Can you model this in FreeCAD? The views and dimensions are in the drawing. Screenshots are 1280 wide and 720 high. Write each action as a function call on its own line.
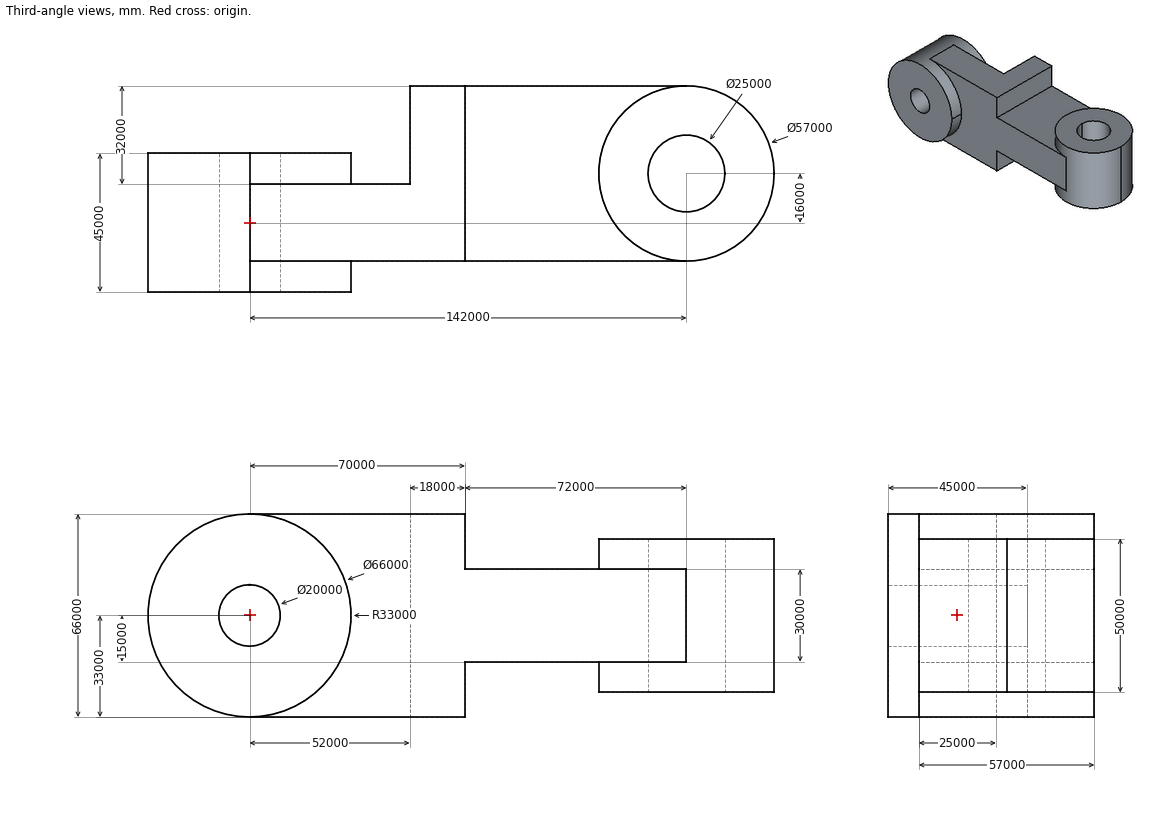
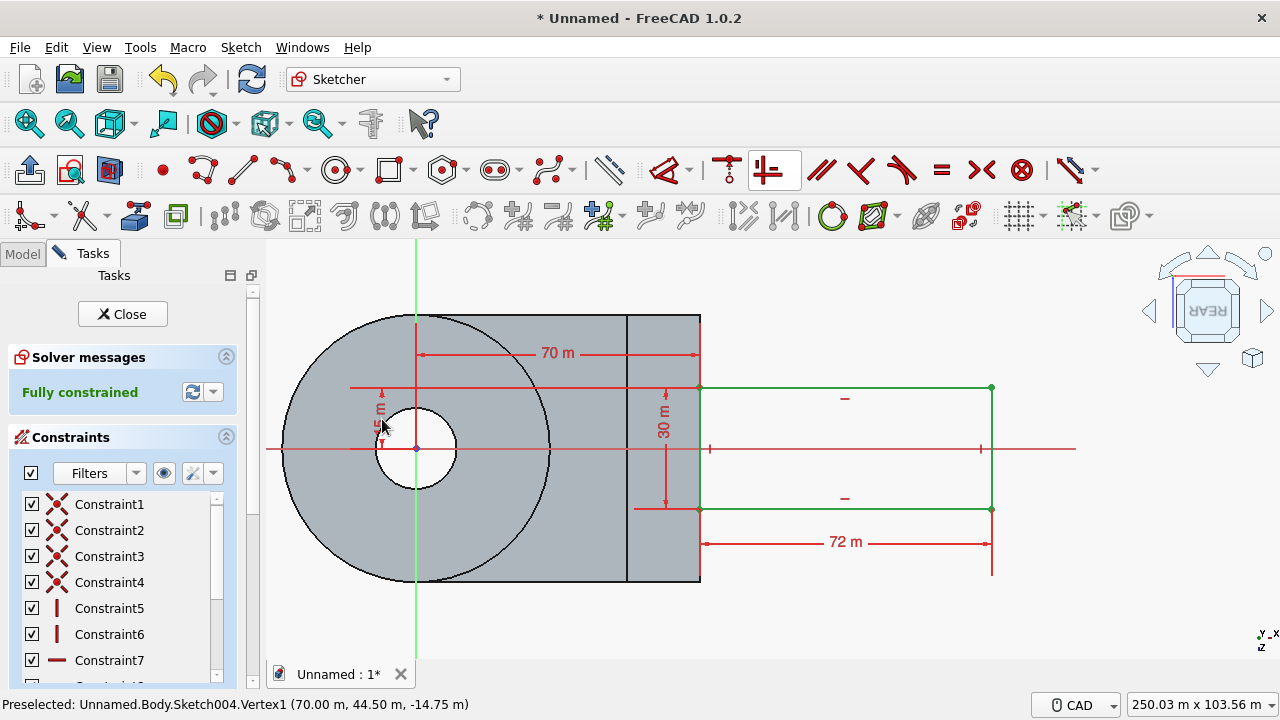
click(123, 314)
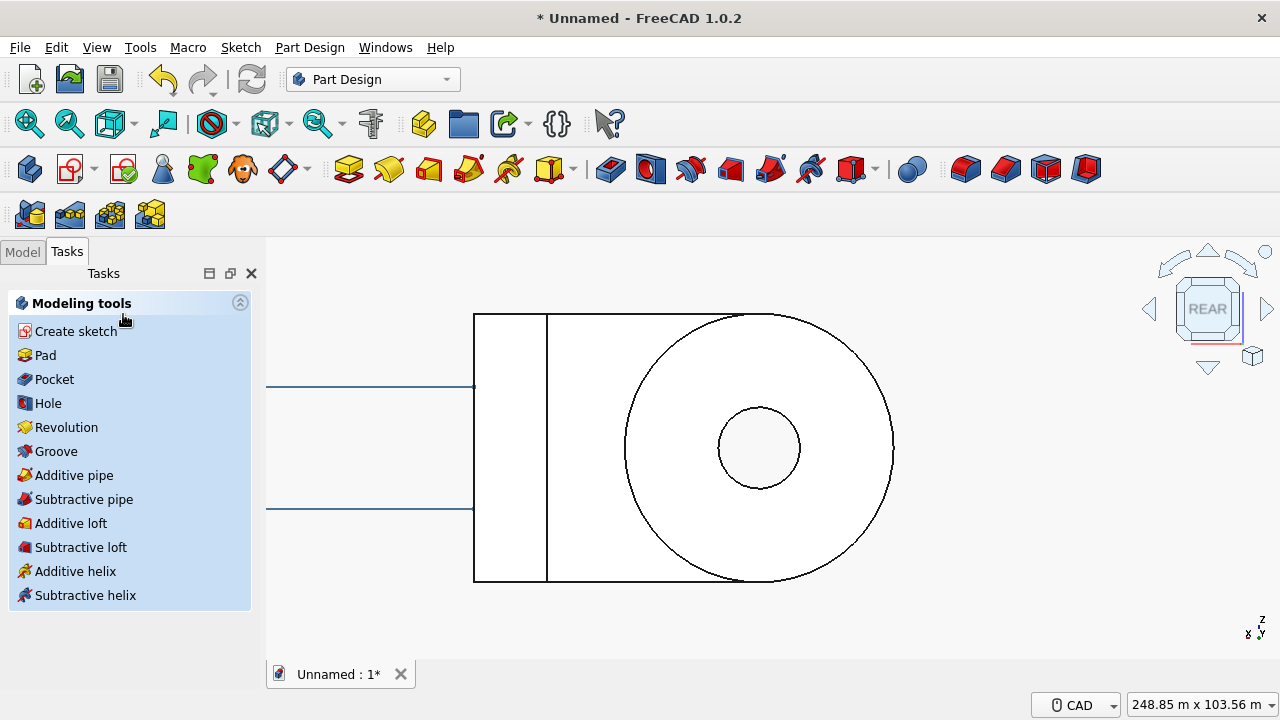
click(350, 170)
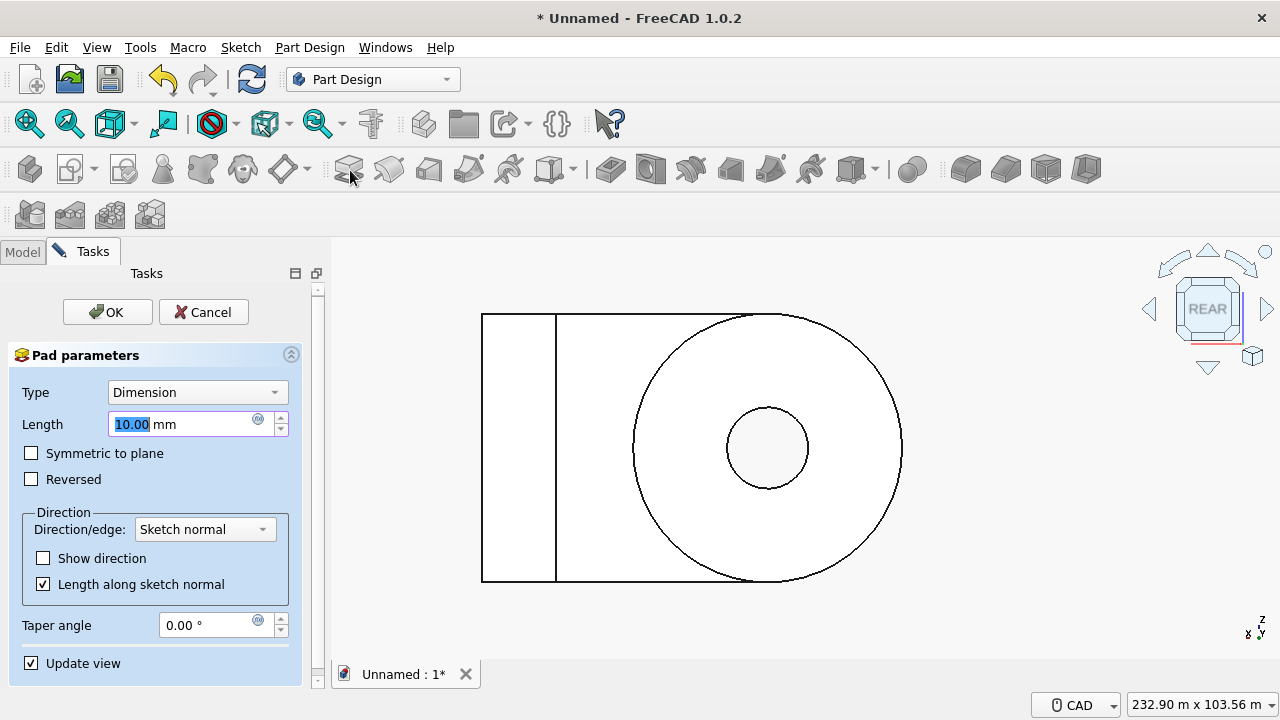
text(57000)
key(Tab)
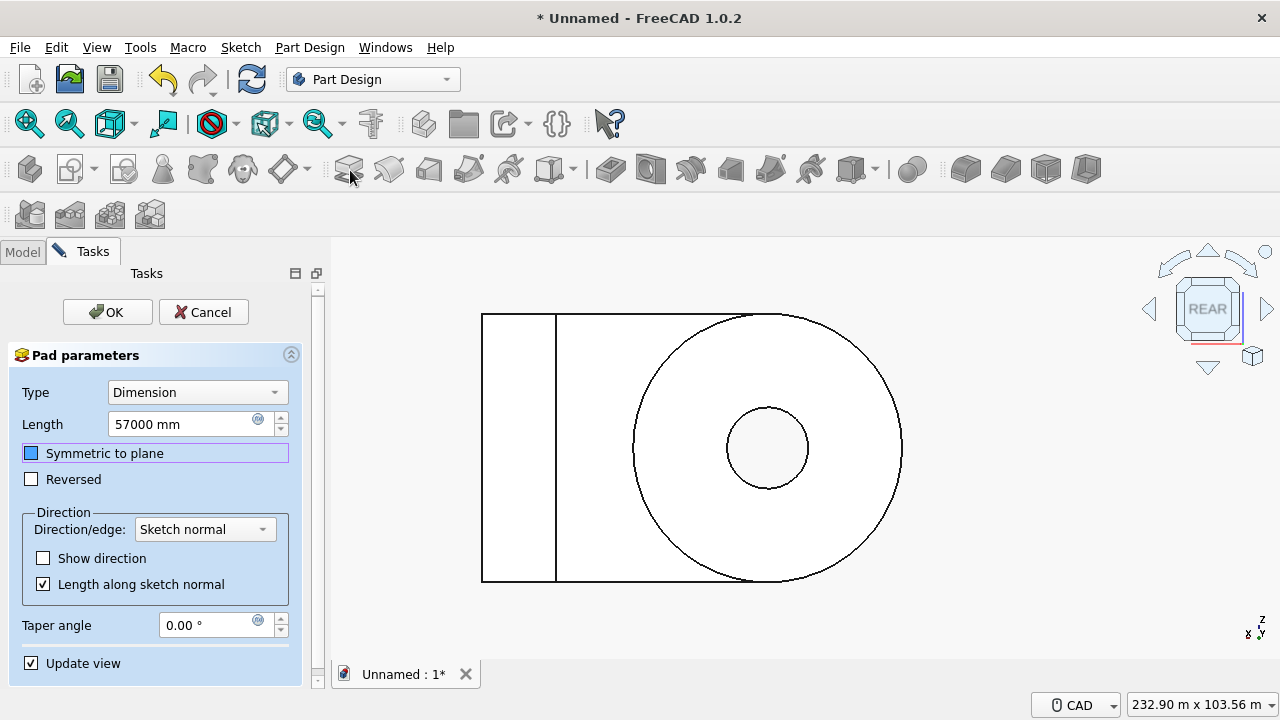
click(30, 479)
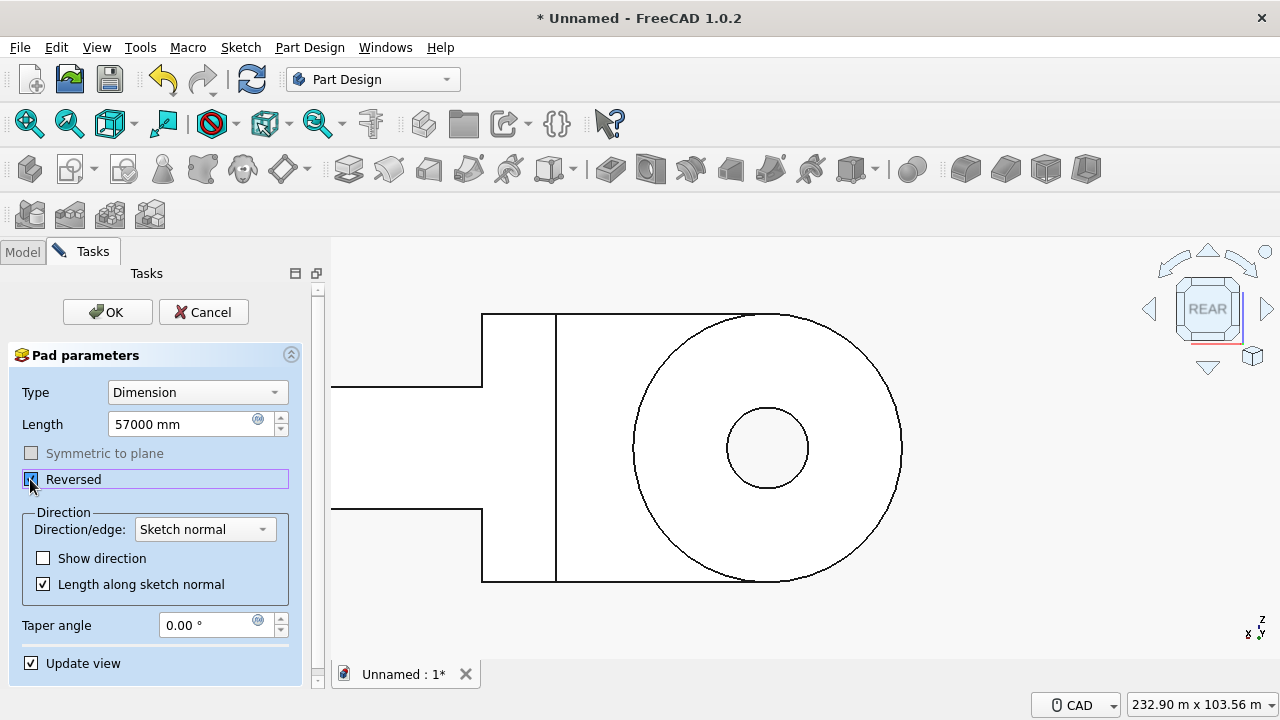
click(108, 312)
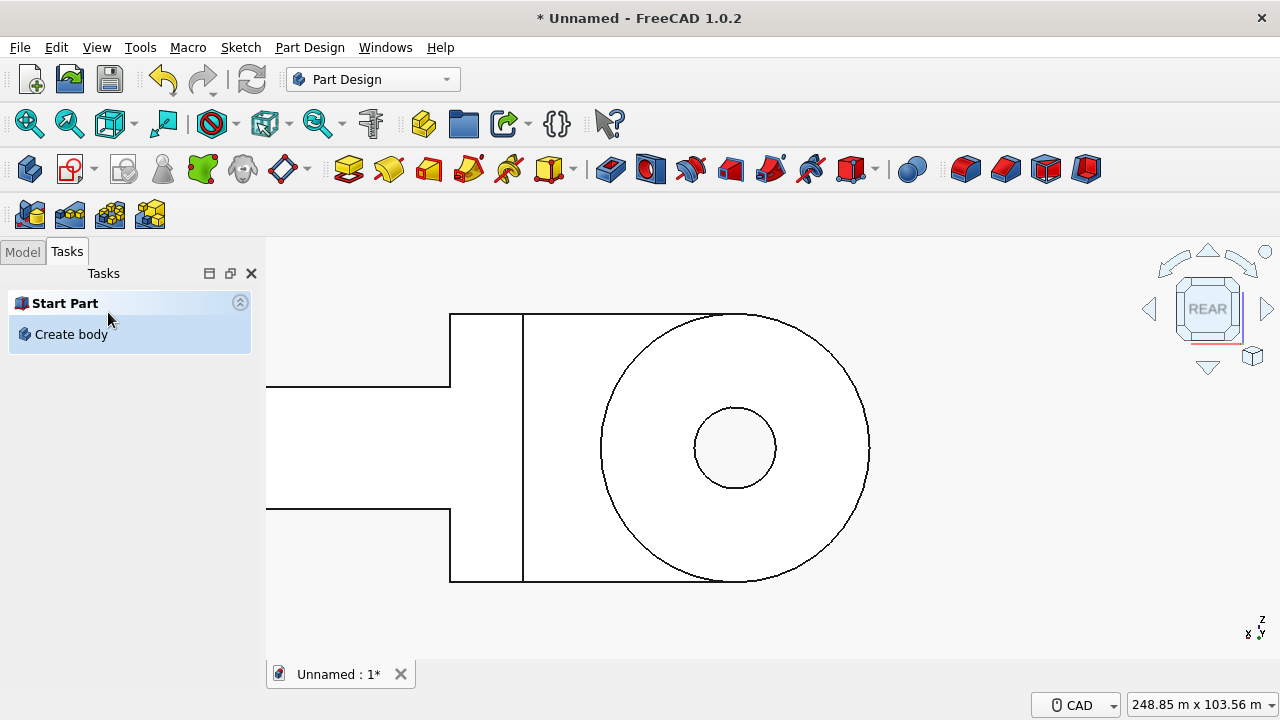
click(30, 124)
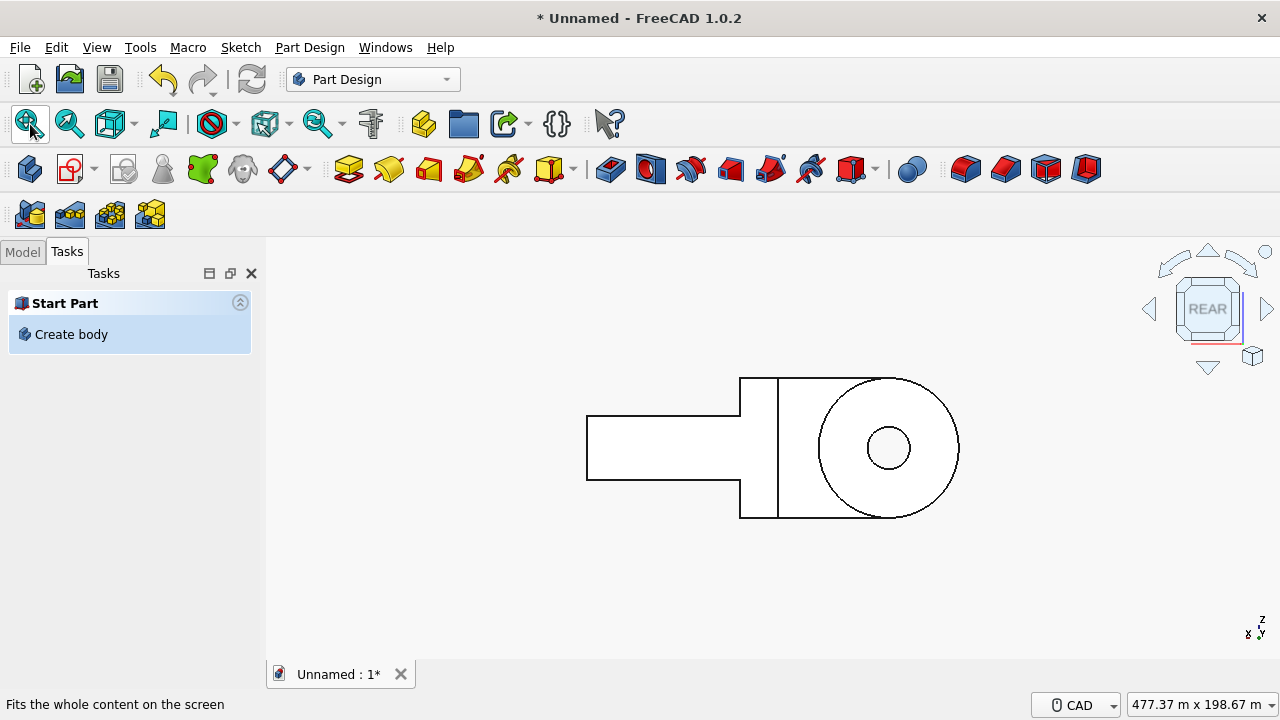
click(70, 170)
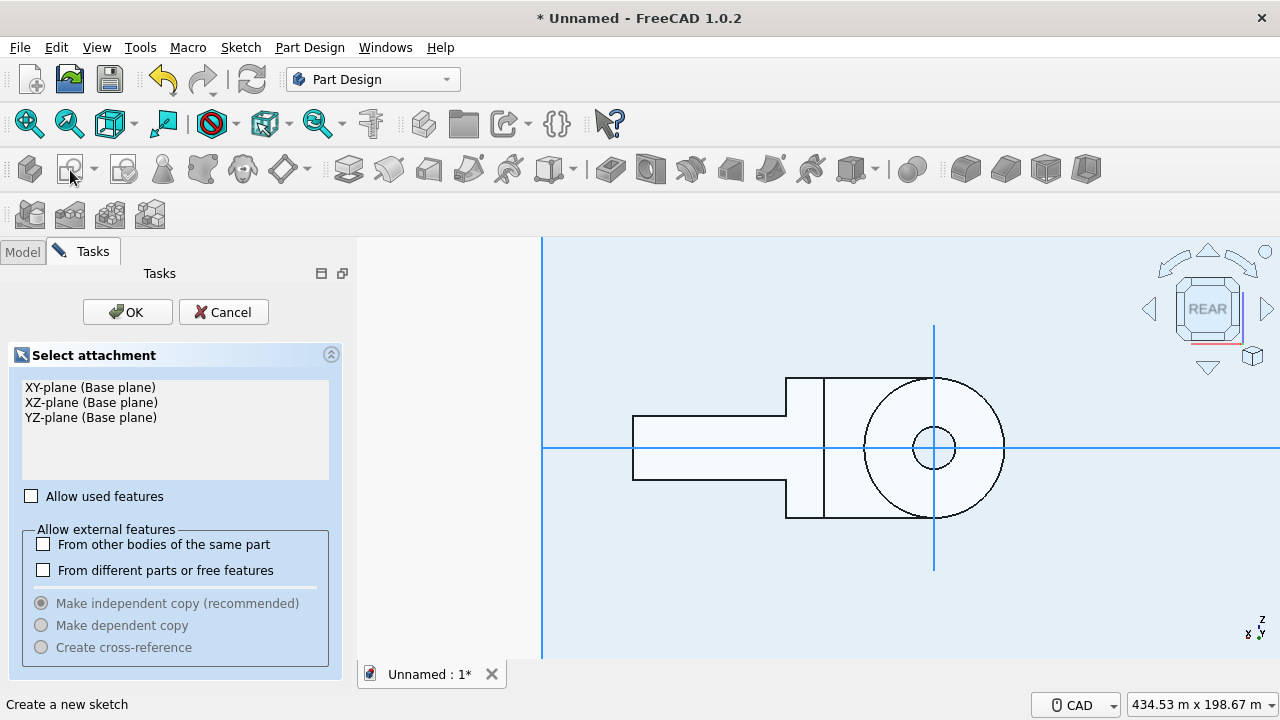
click(82, 388)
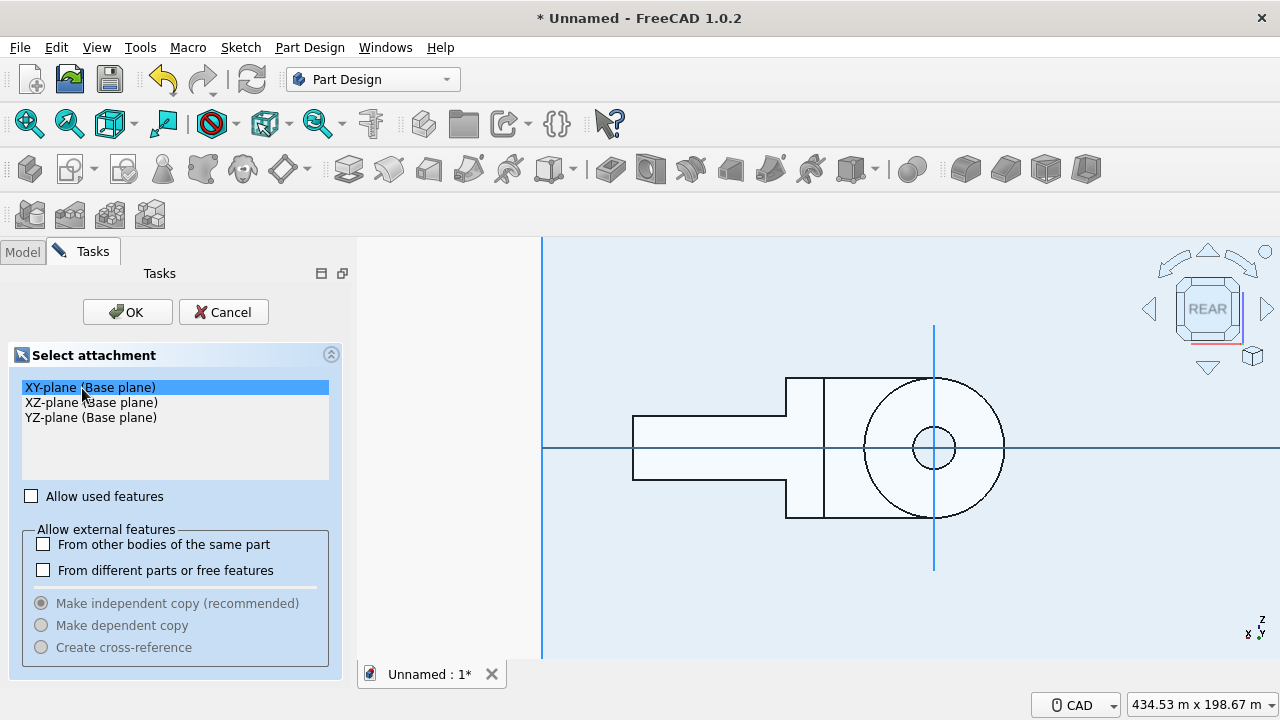
click(128, 312)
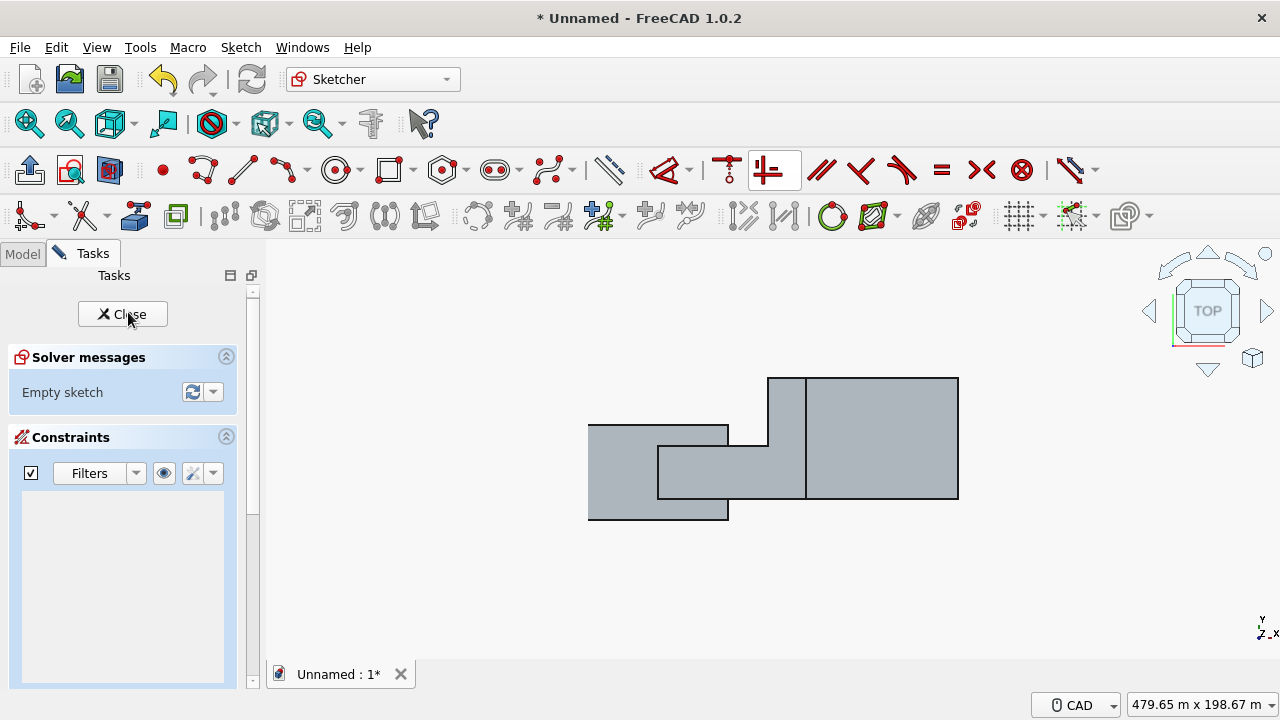
click(110, 170)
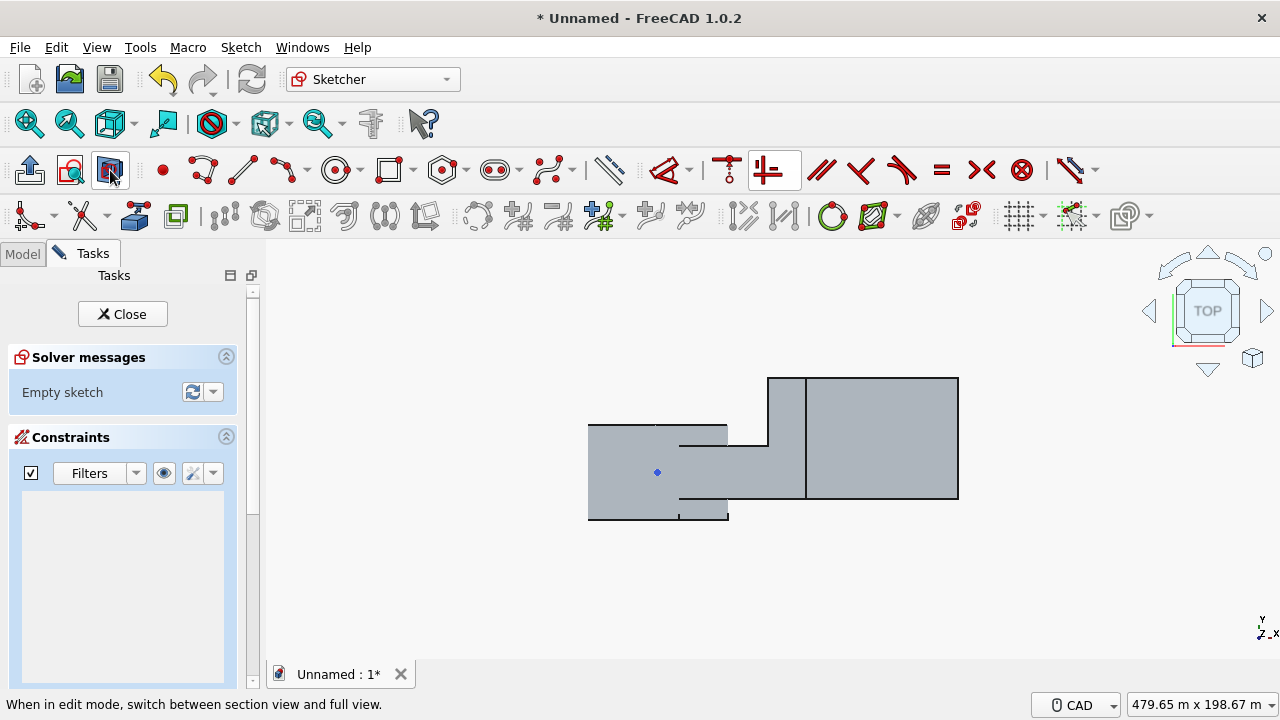
scroll(1115, 430, up, 4)